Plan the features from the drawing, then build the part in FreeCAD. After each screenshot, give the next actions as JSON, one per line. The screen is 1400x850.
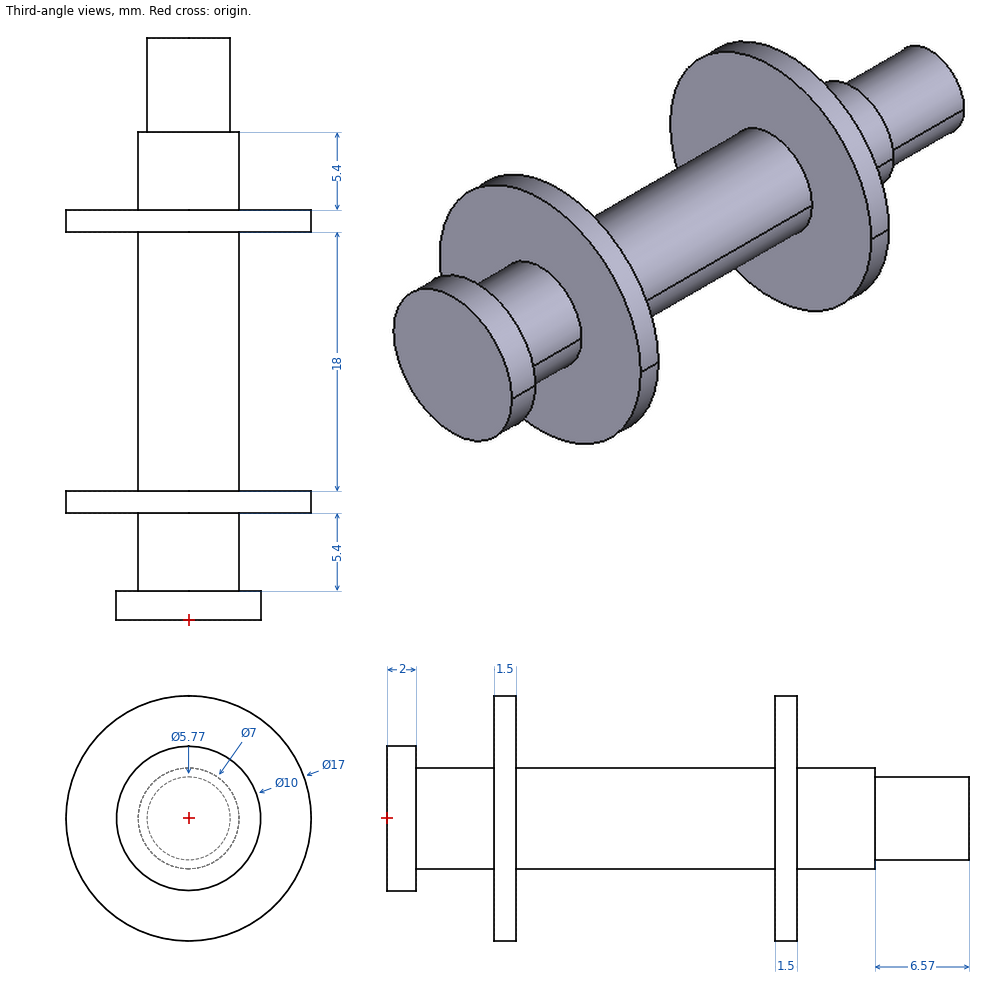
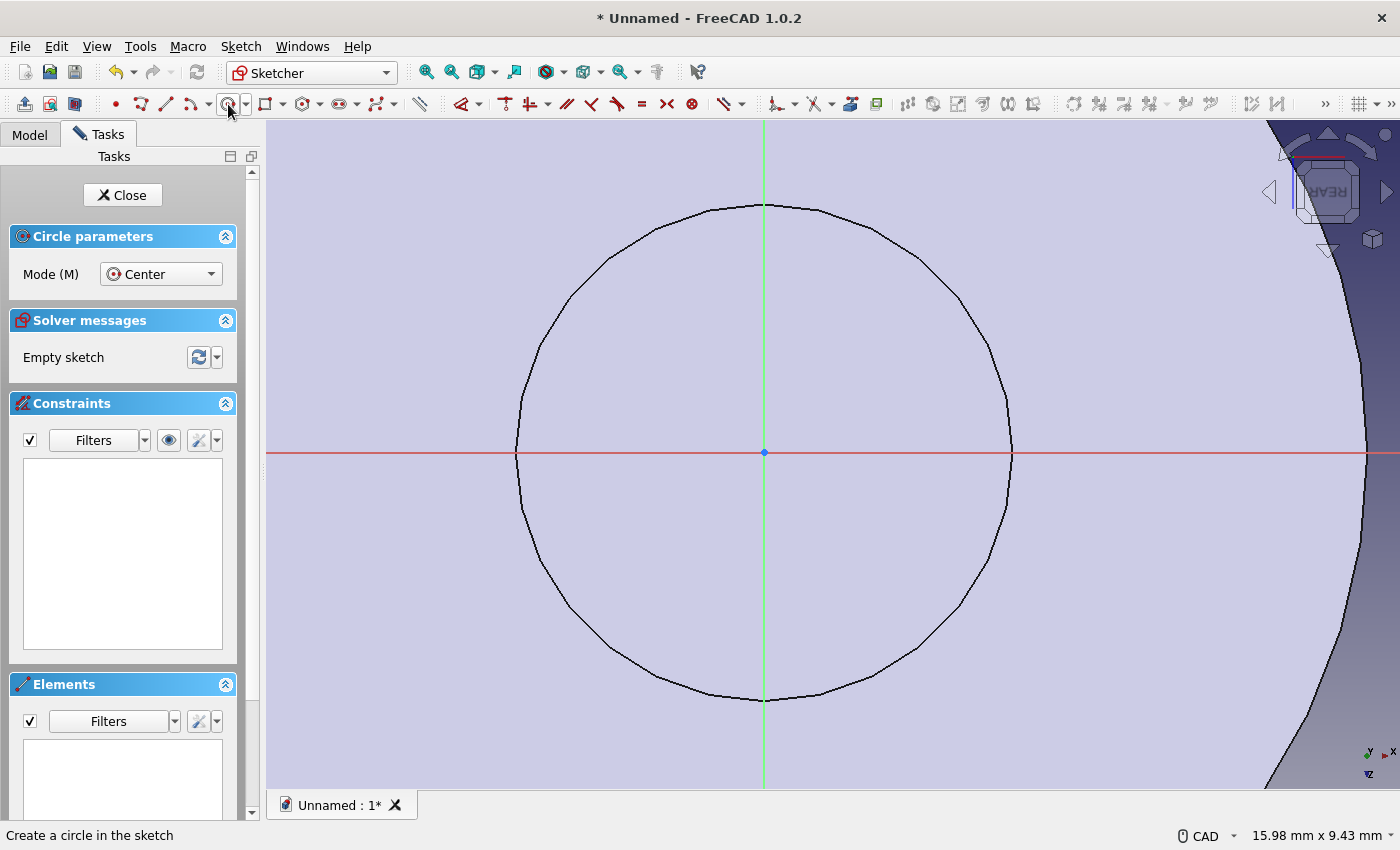
{"action": "left_click", "coordinate": [764, 453]}
{"action": "left_click", "coordinate": [909, 308]}
{"action": "key", "text": "Escape"}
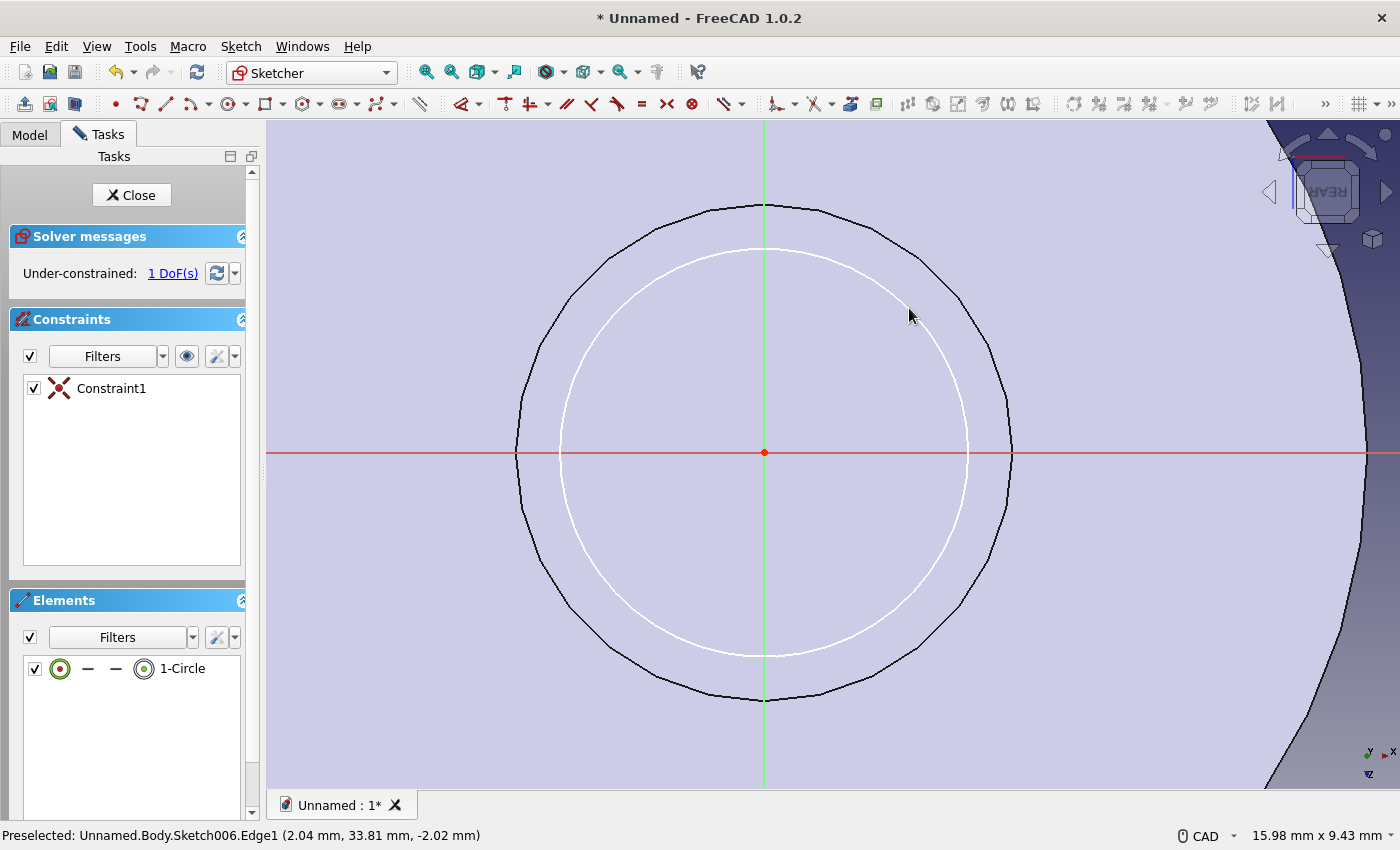
{"action": "left_click", "coordinate": [460, 104]}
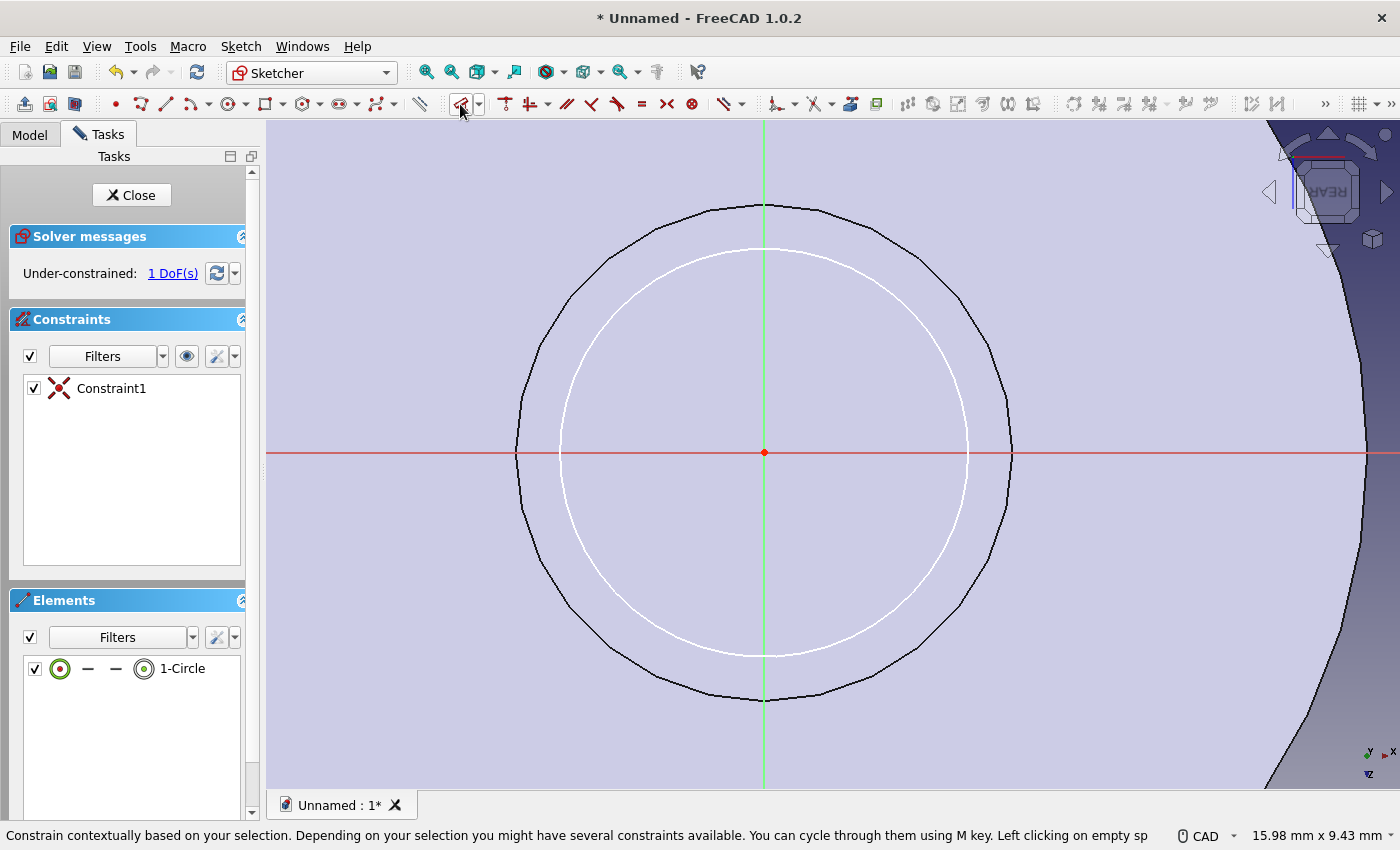
{"action": "left_click", "coordinate": [908, 308]}
{"action": "left_click", "coordinate": [931, 285]}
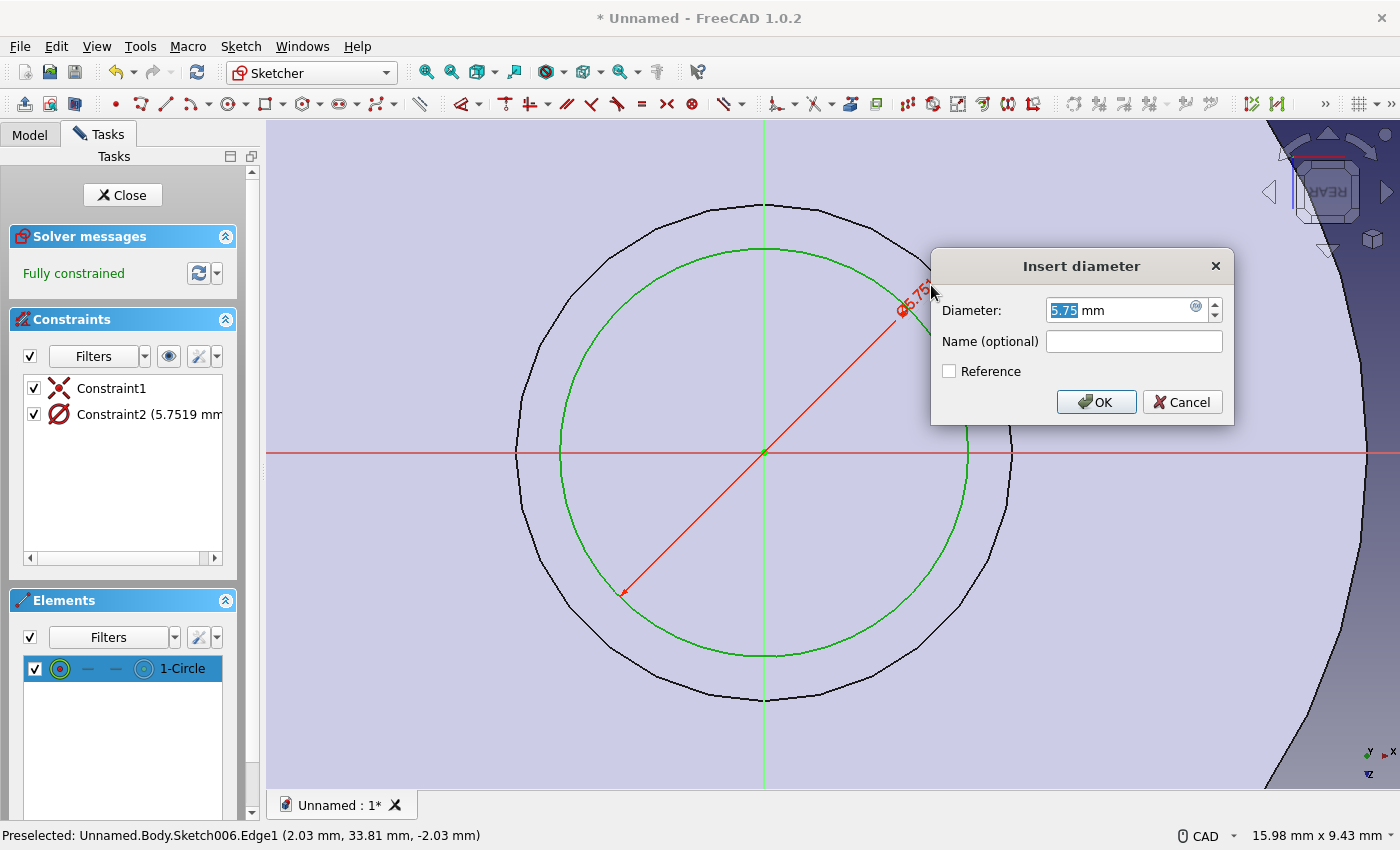
{"action": "type", "text": "5.77"}
{"action": "key", "text": "Return"}
{"action": "key", "text": "Escape"}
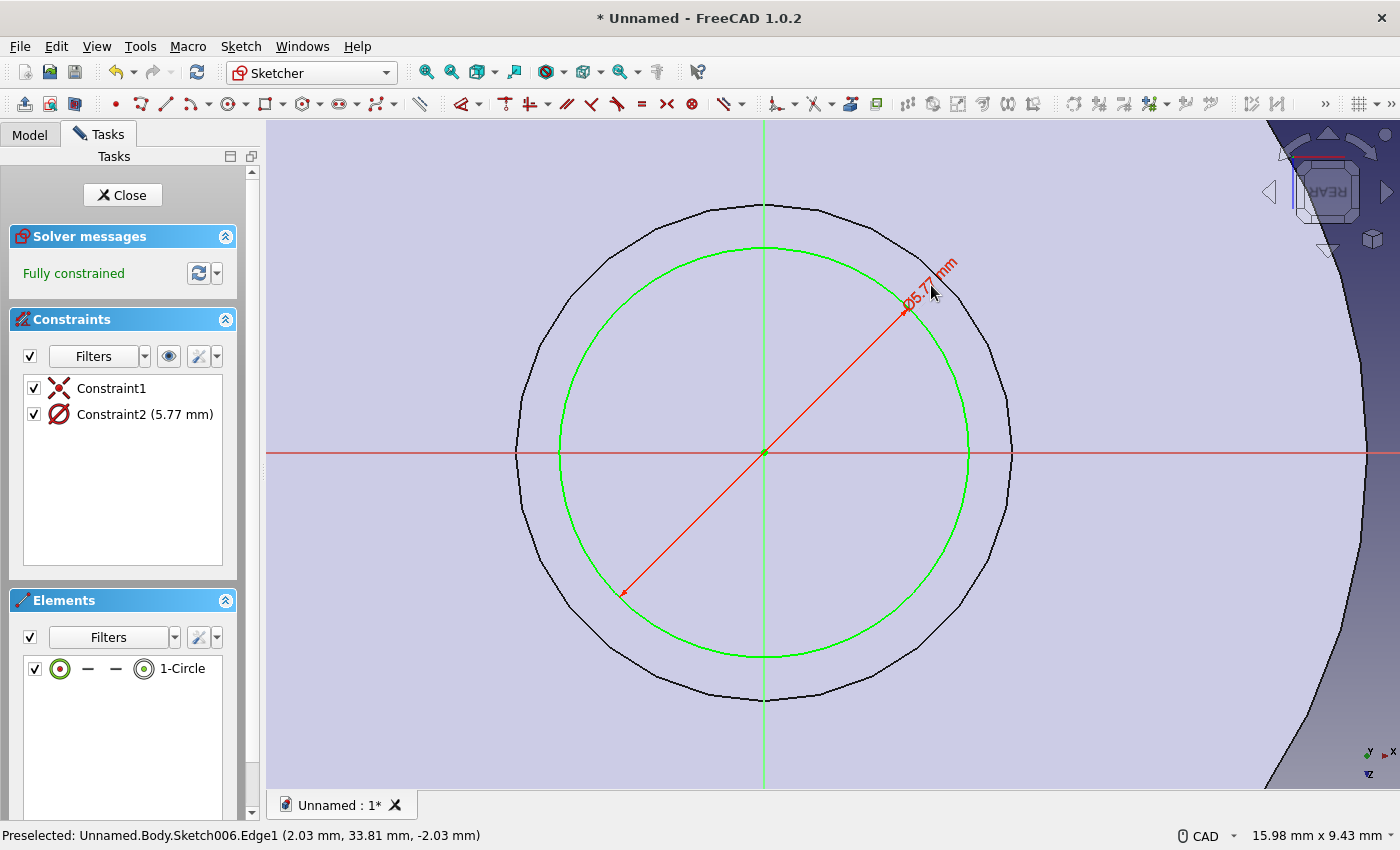
{"action": "left_click", "coordinate": [123, 195]}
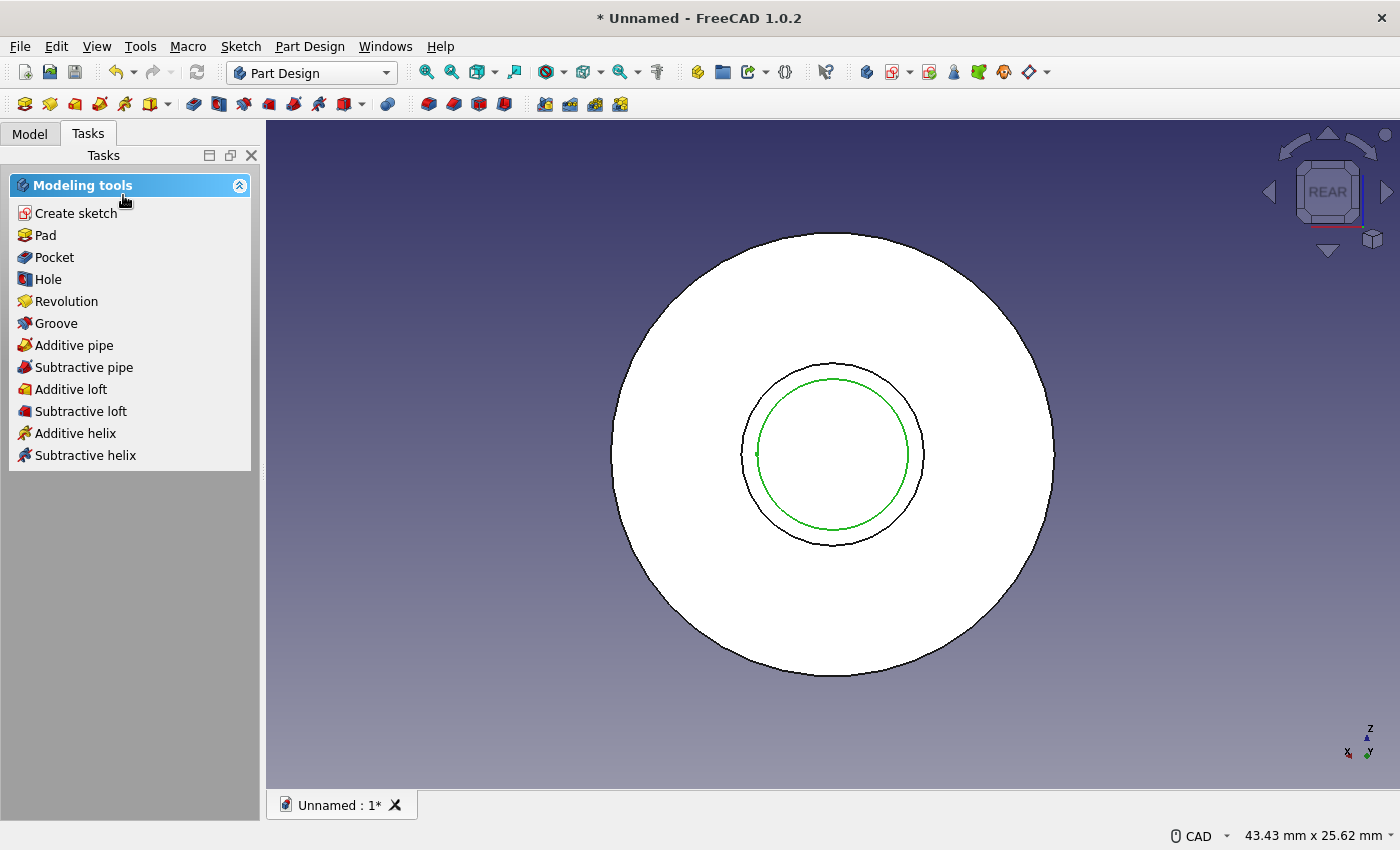
{"action": "left_click", "coordinate": [25, 104]}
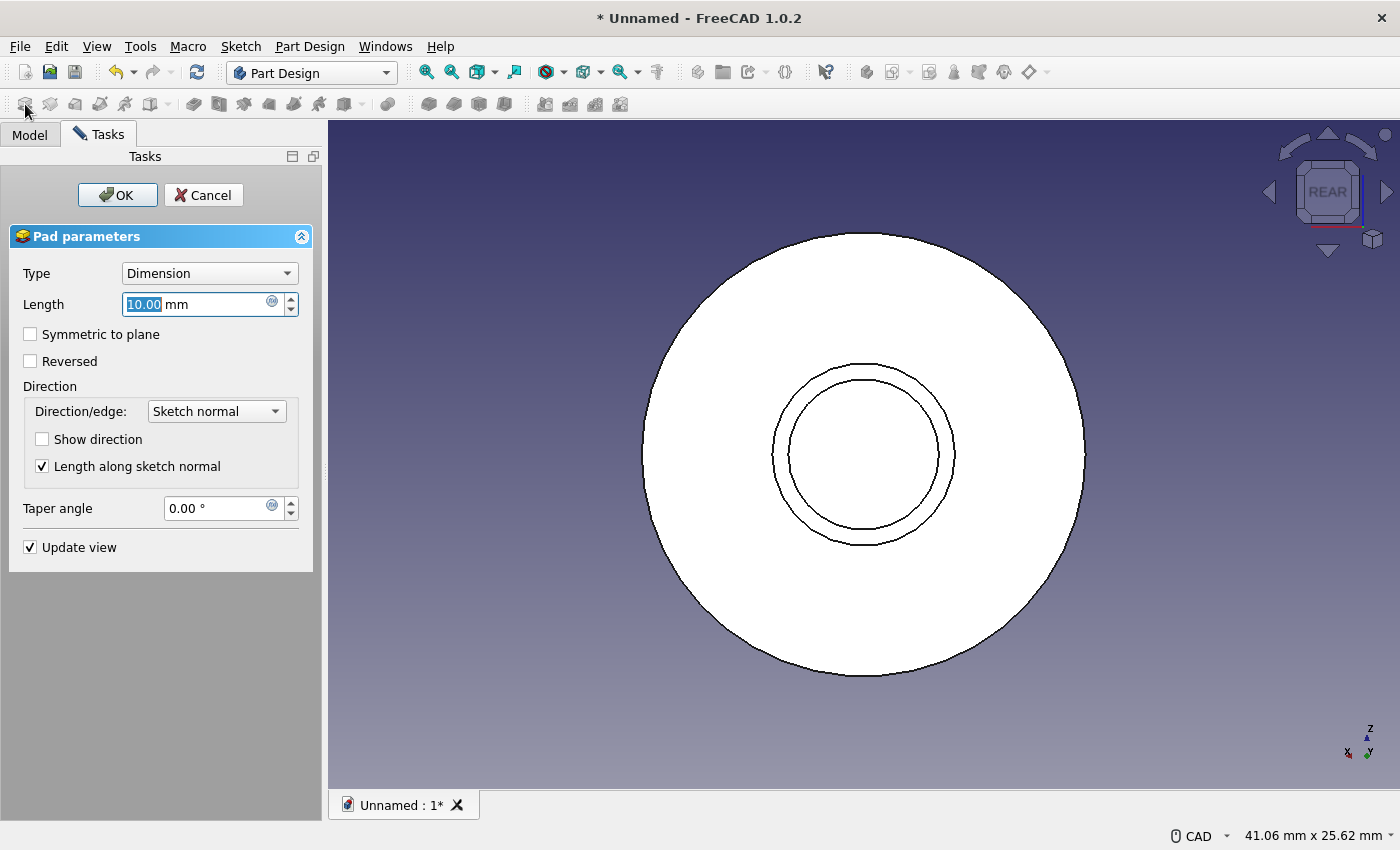
{"action": "type", "text": "6.57"}
{"action": "key", "text": "Tab"}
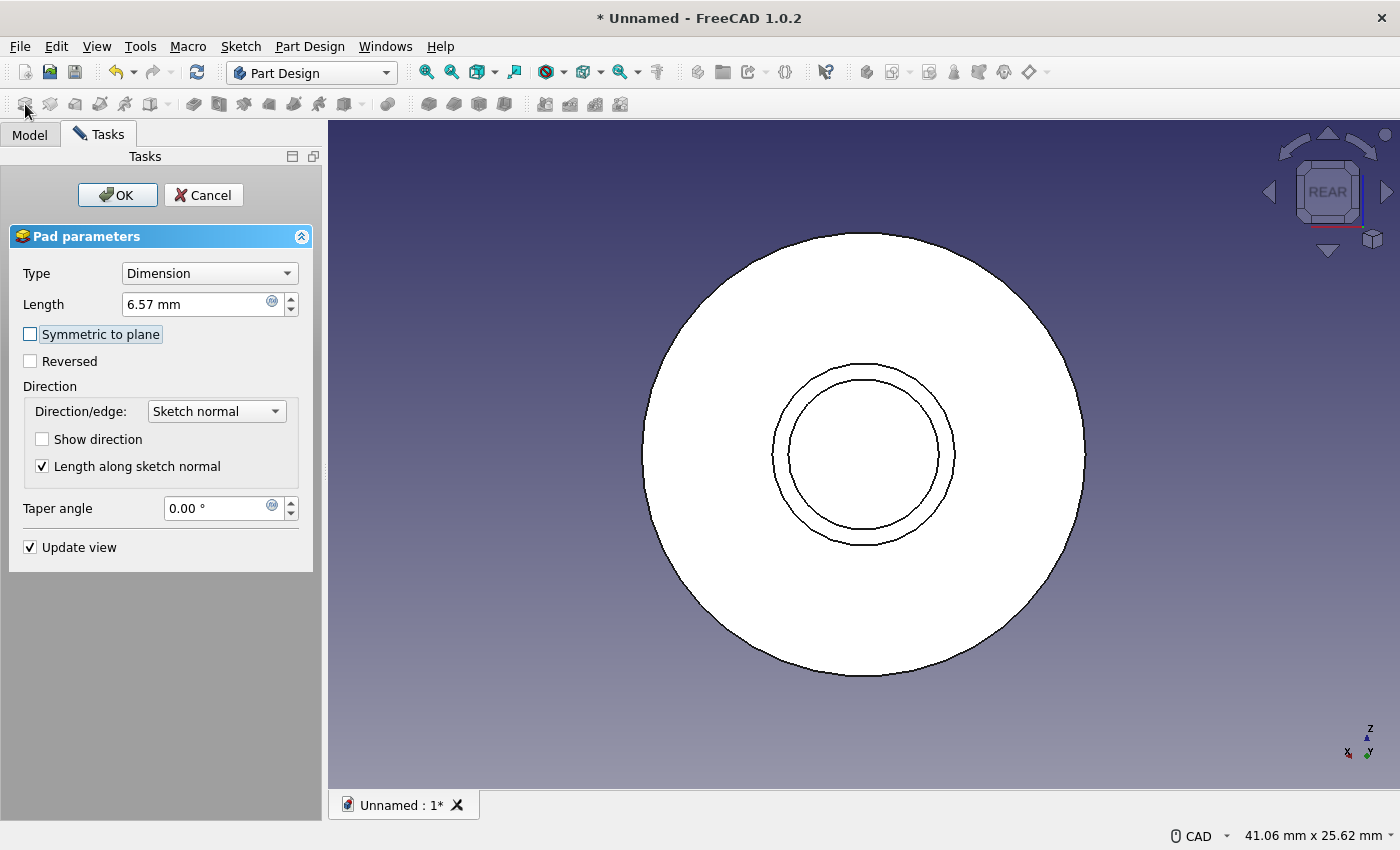
{"action": "left_click", "coordinate": [118, 195]}